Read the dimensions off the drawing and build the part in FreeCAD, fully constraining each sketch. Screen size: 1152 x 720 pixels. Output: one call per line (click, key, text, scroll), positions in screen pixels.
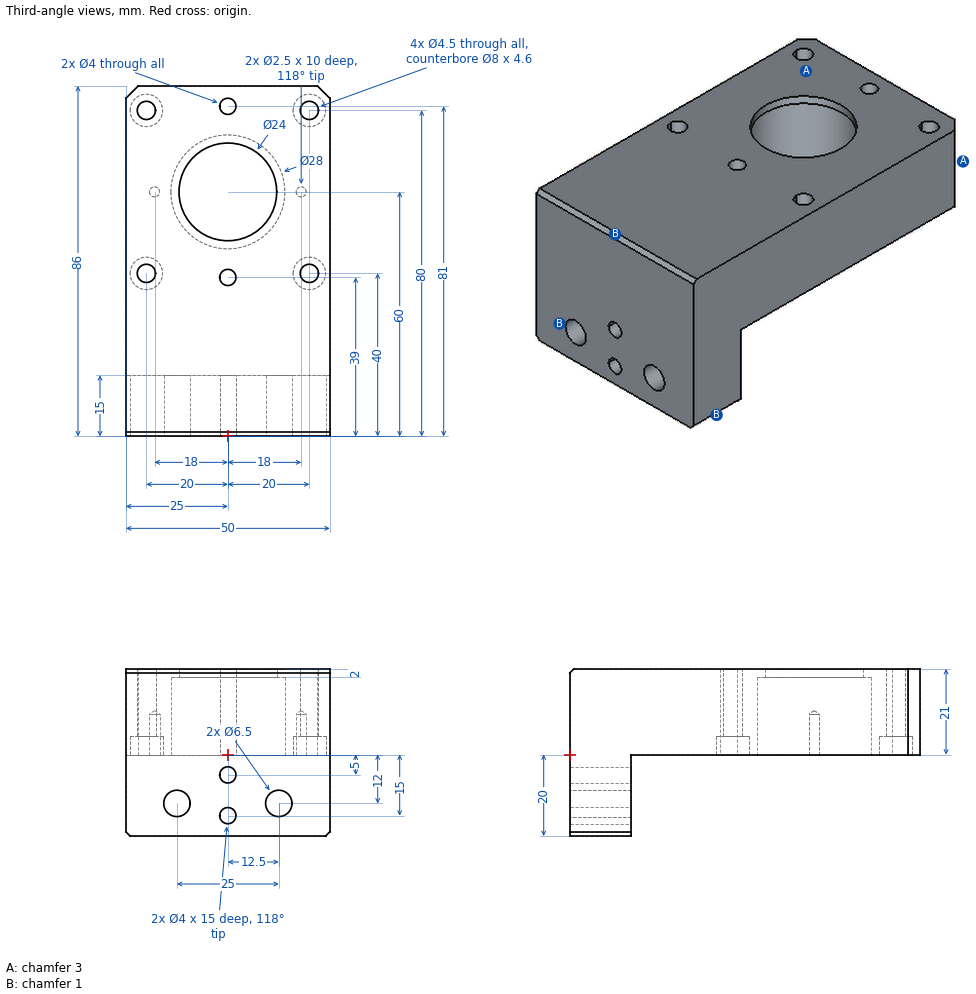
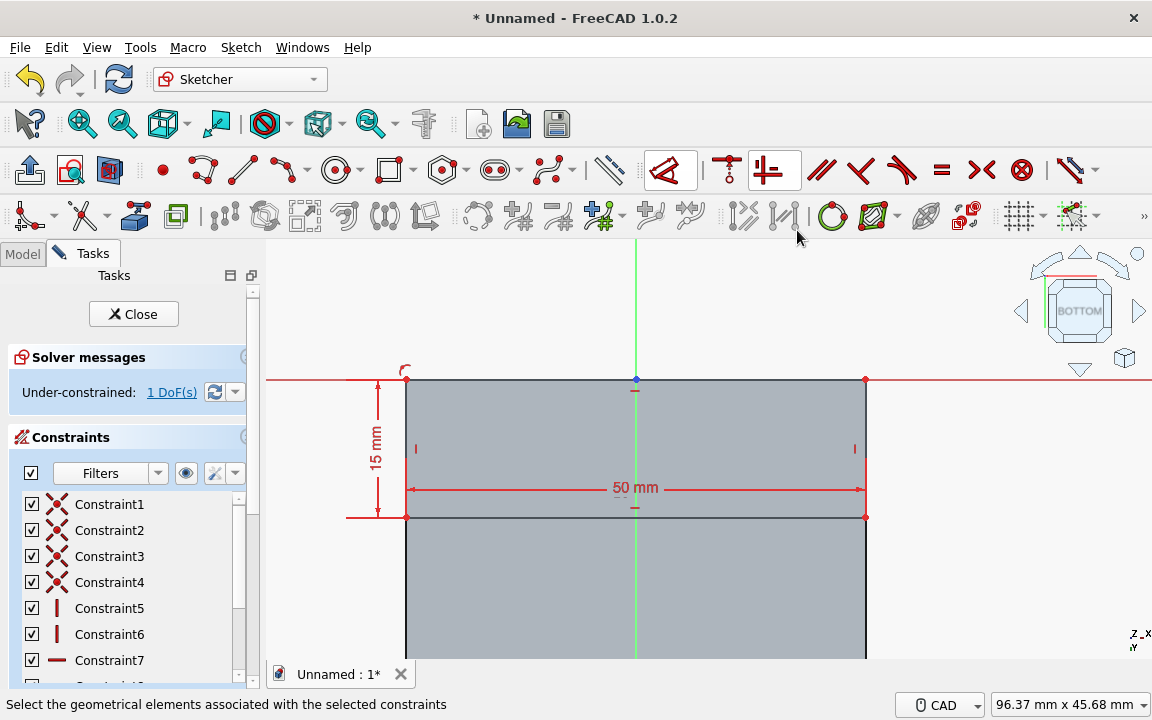
click(406, 380)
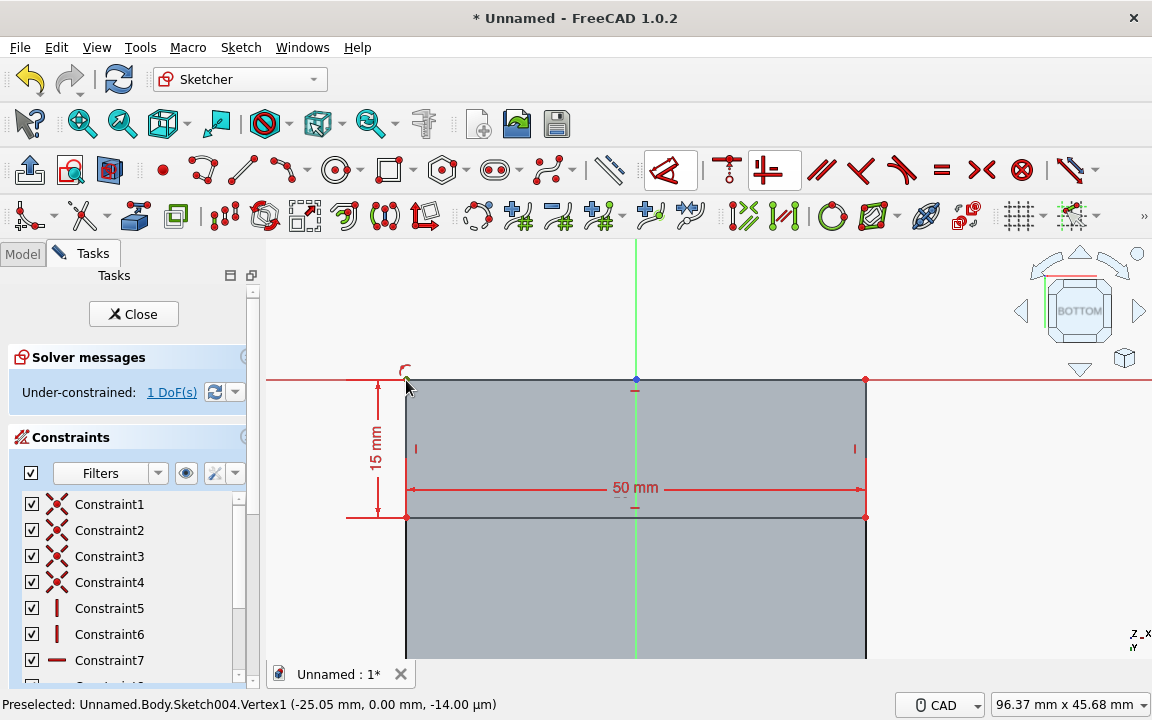
key(l)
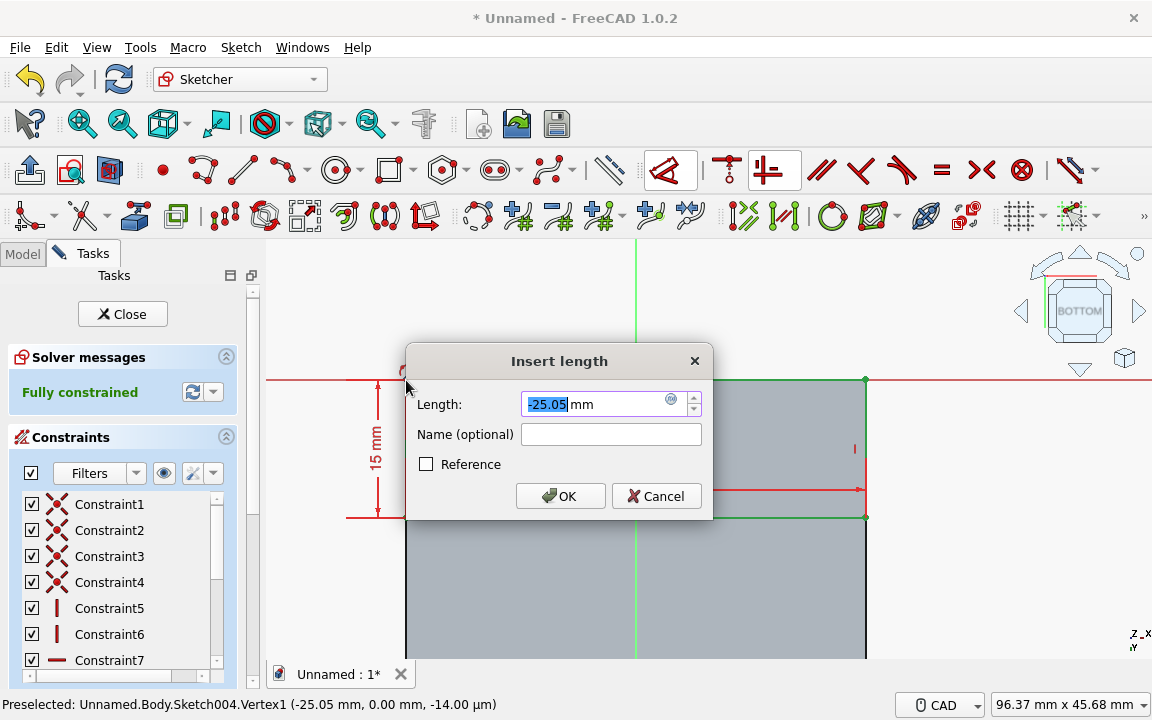
text(-25)
key(Return)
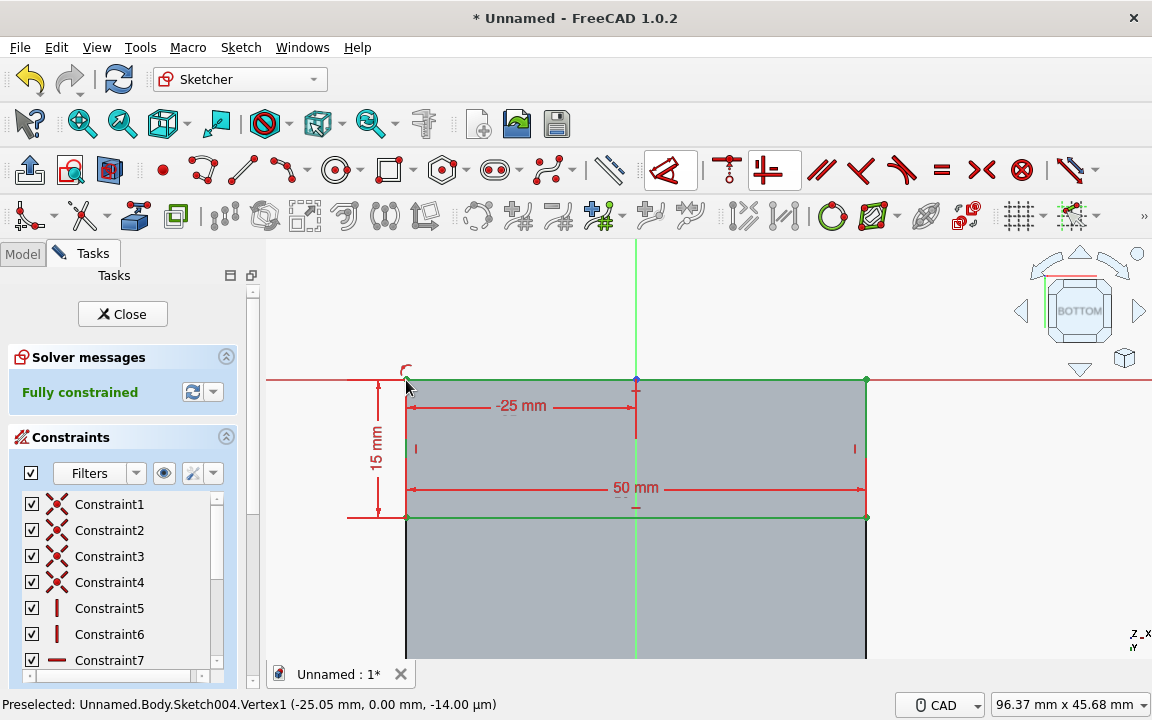
click(123, 314)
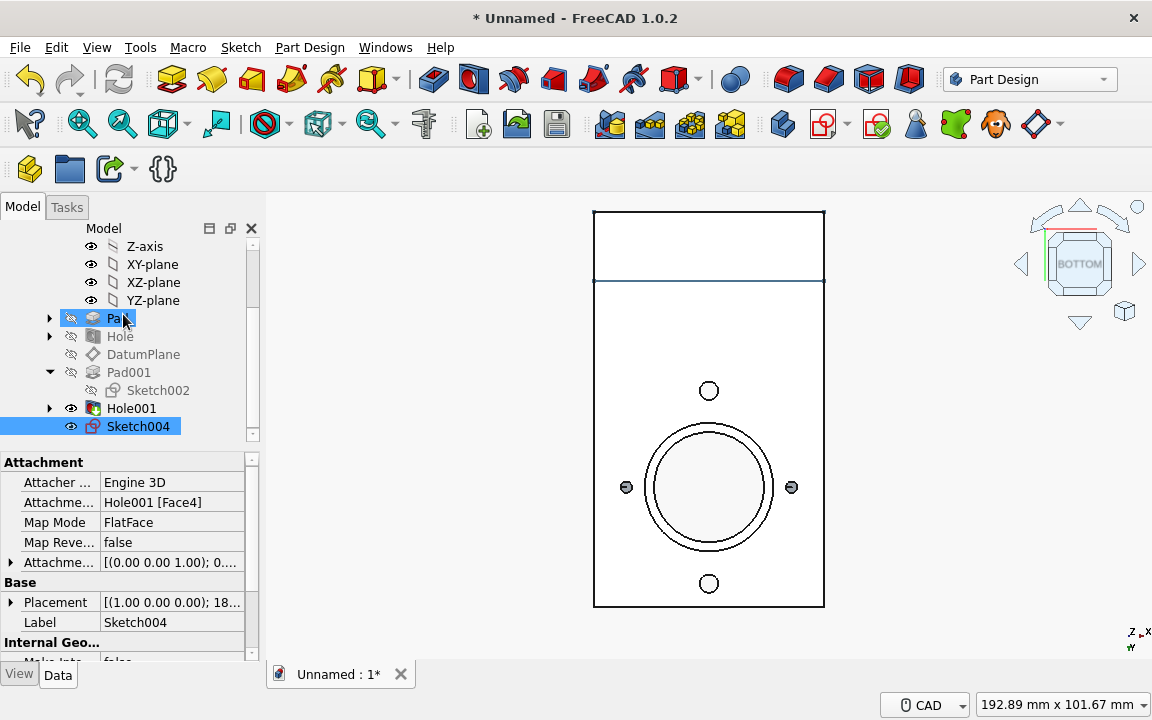
click(172, 80)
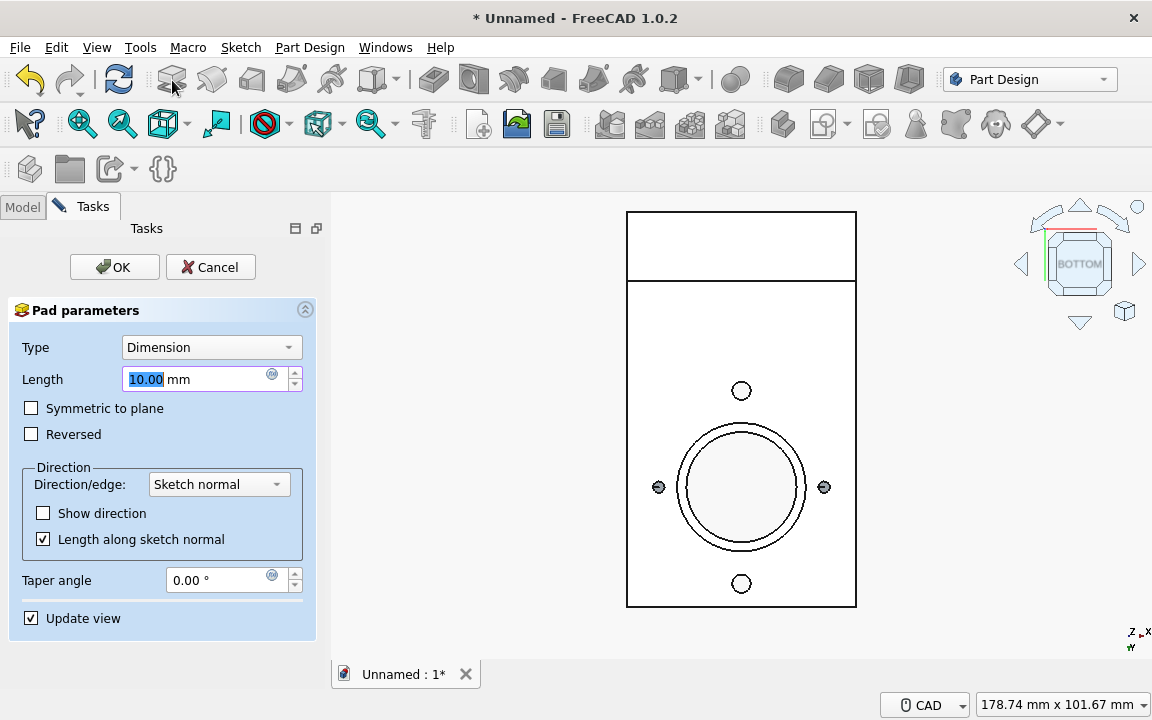
text(20)
key(Tab)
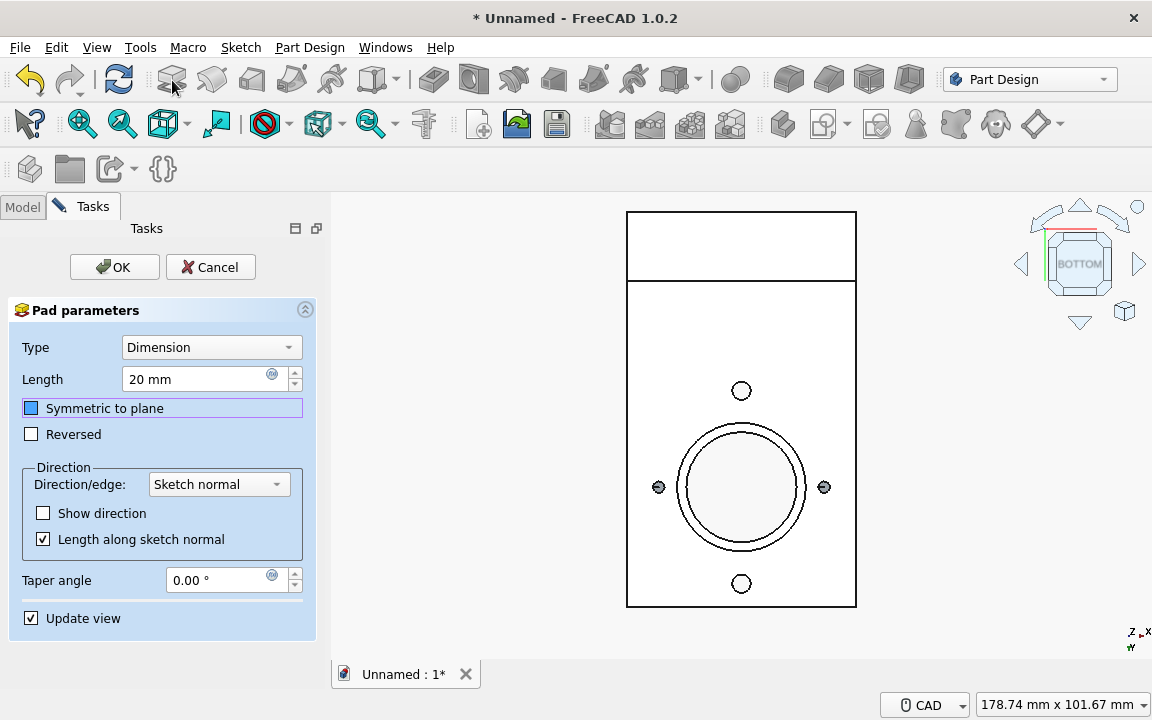
click(115, 267)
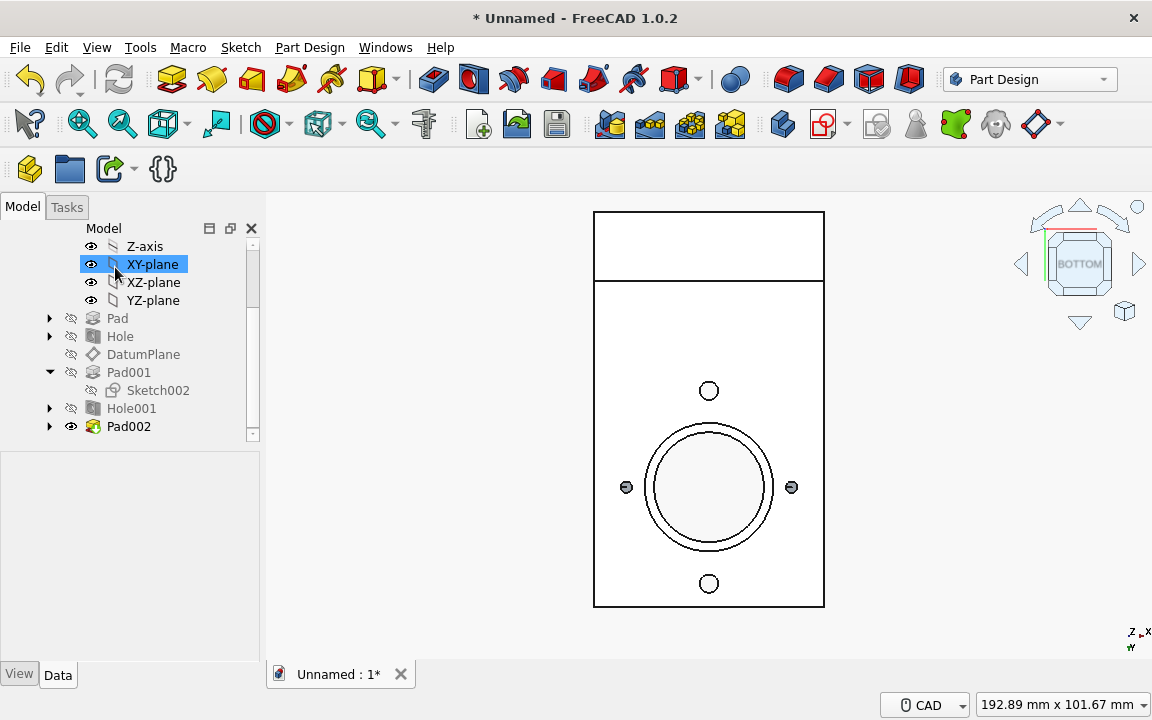
click(824, 124)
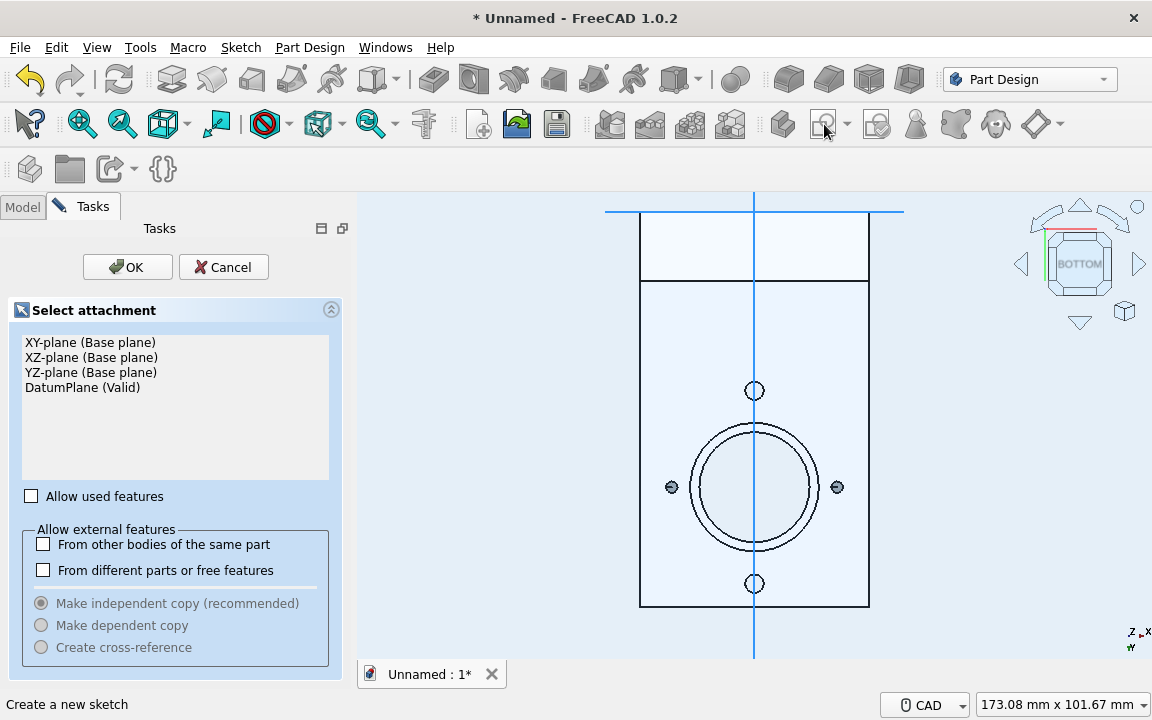
click(82, 358)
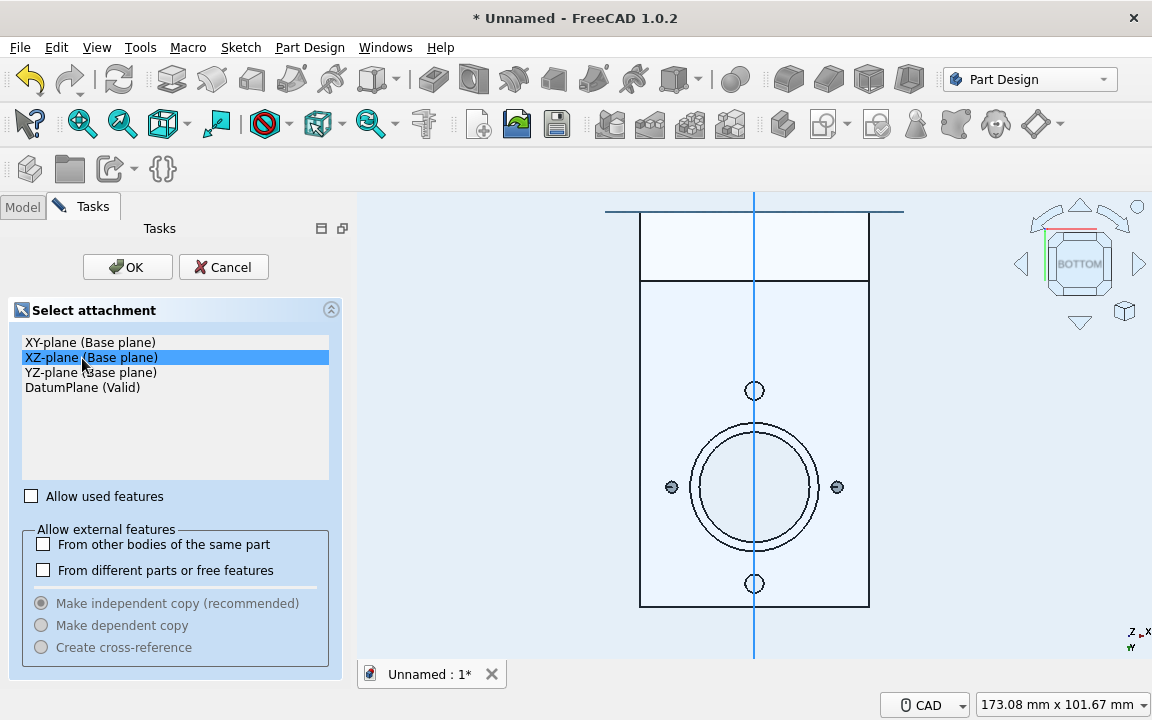
click(128, 267)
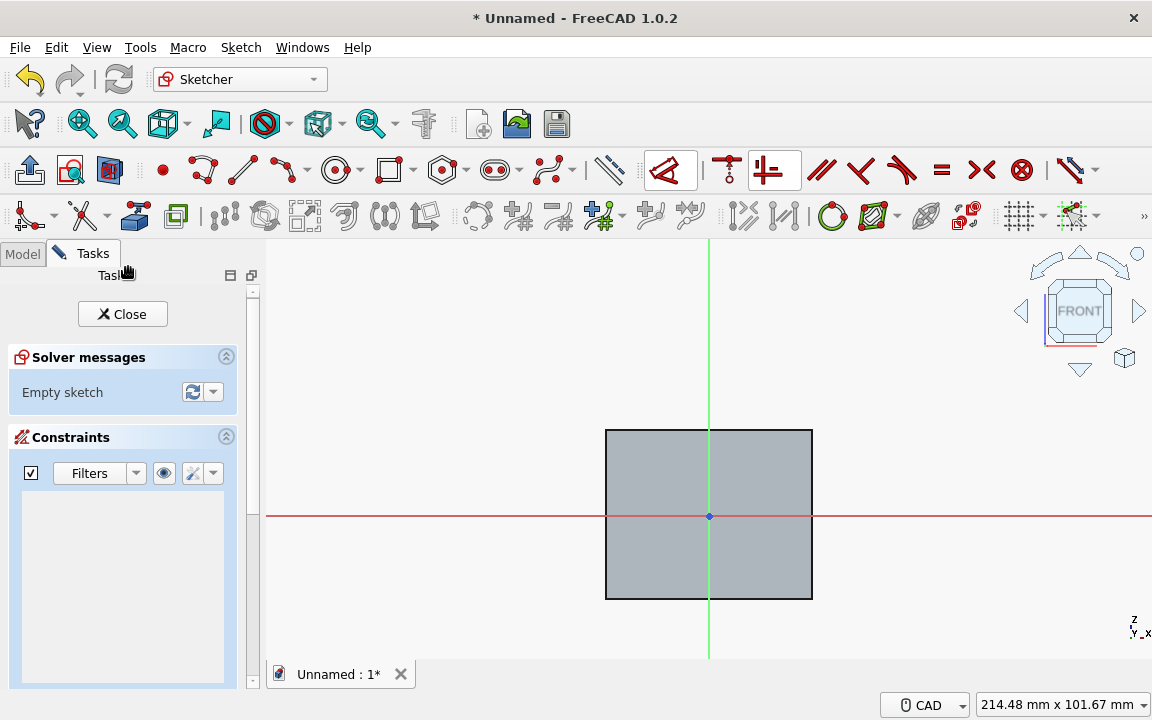
scroll(731, 580, up, 7)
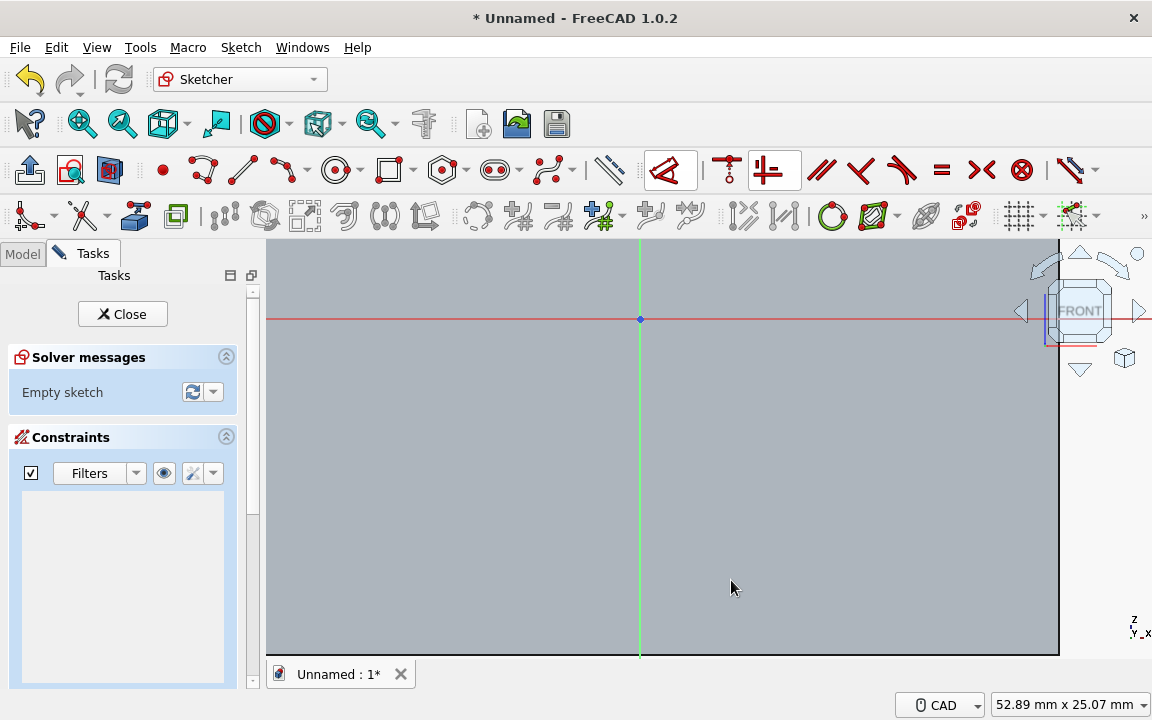
key(g)
key(c)